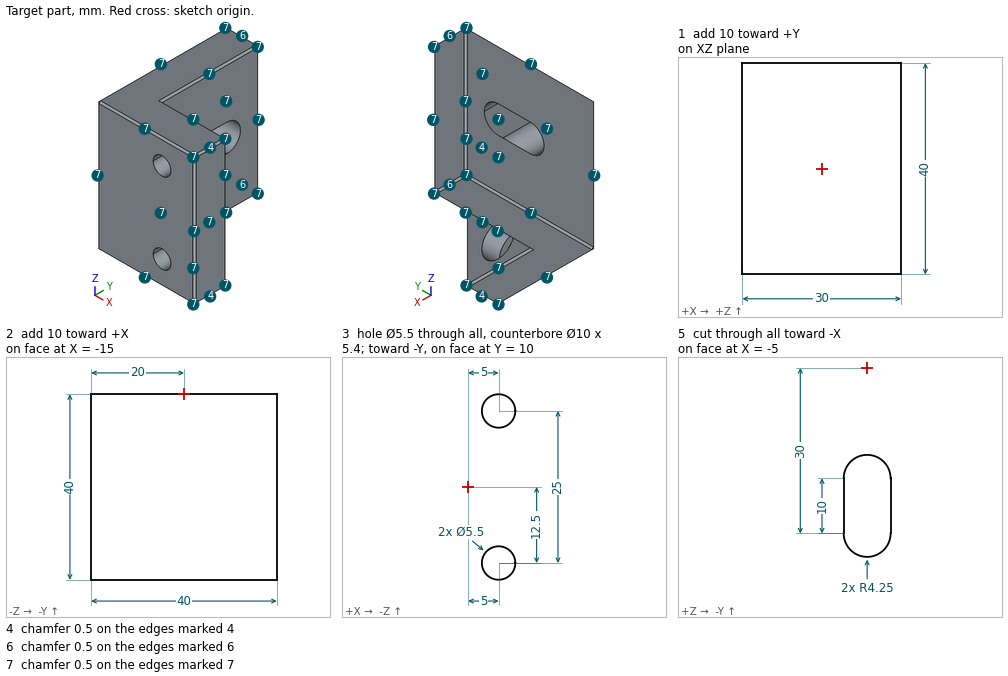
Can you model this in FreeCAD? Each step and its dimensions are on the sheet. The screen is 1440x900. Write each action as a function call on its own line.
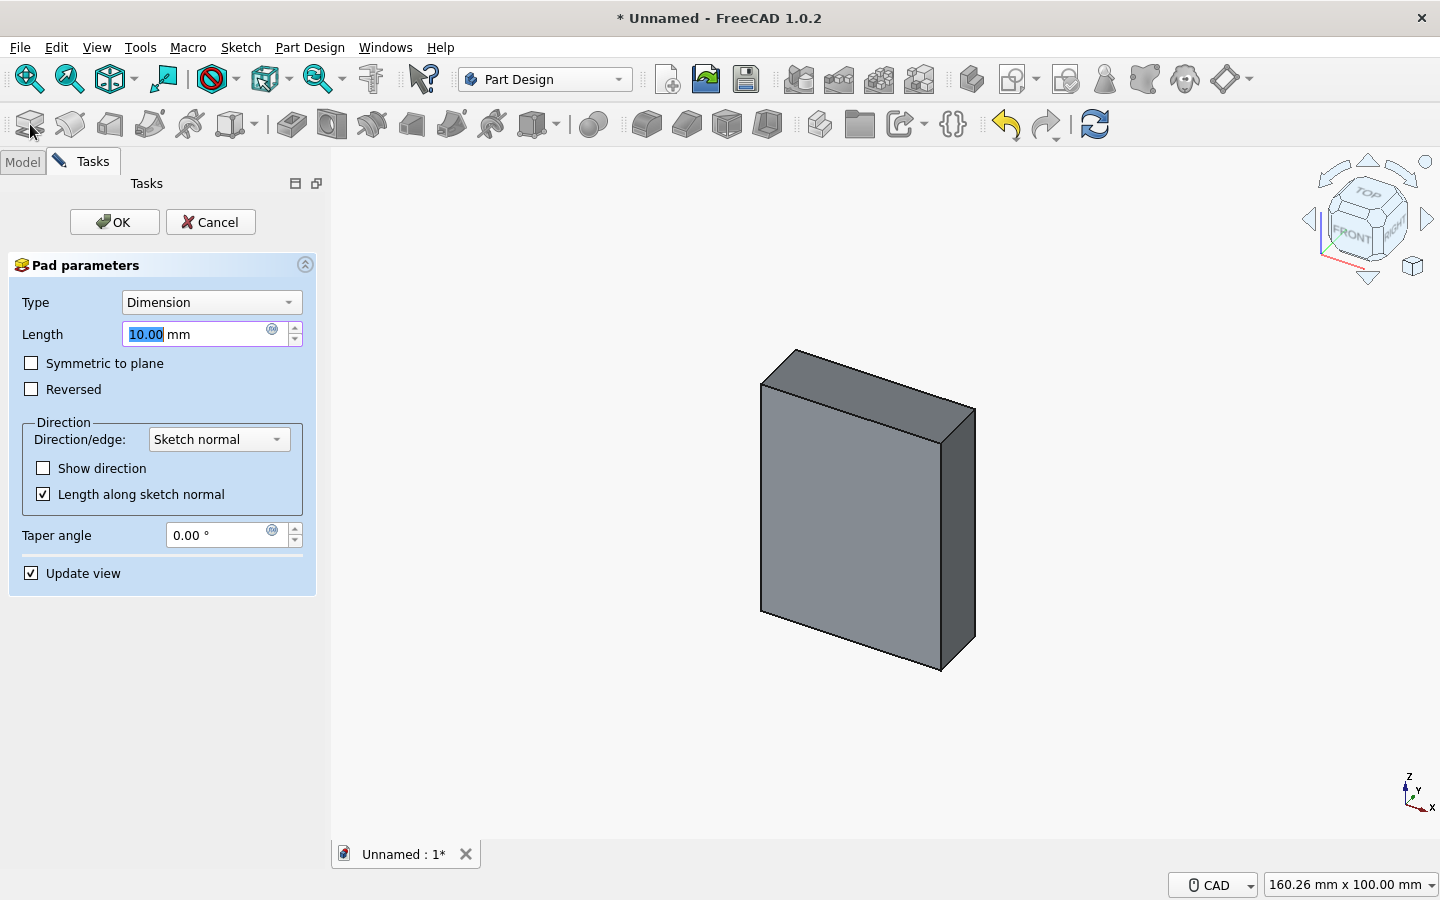
text(10)
key(Tab)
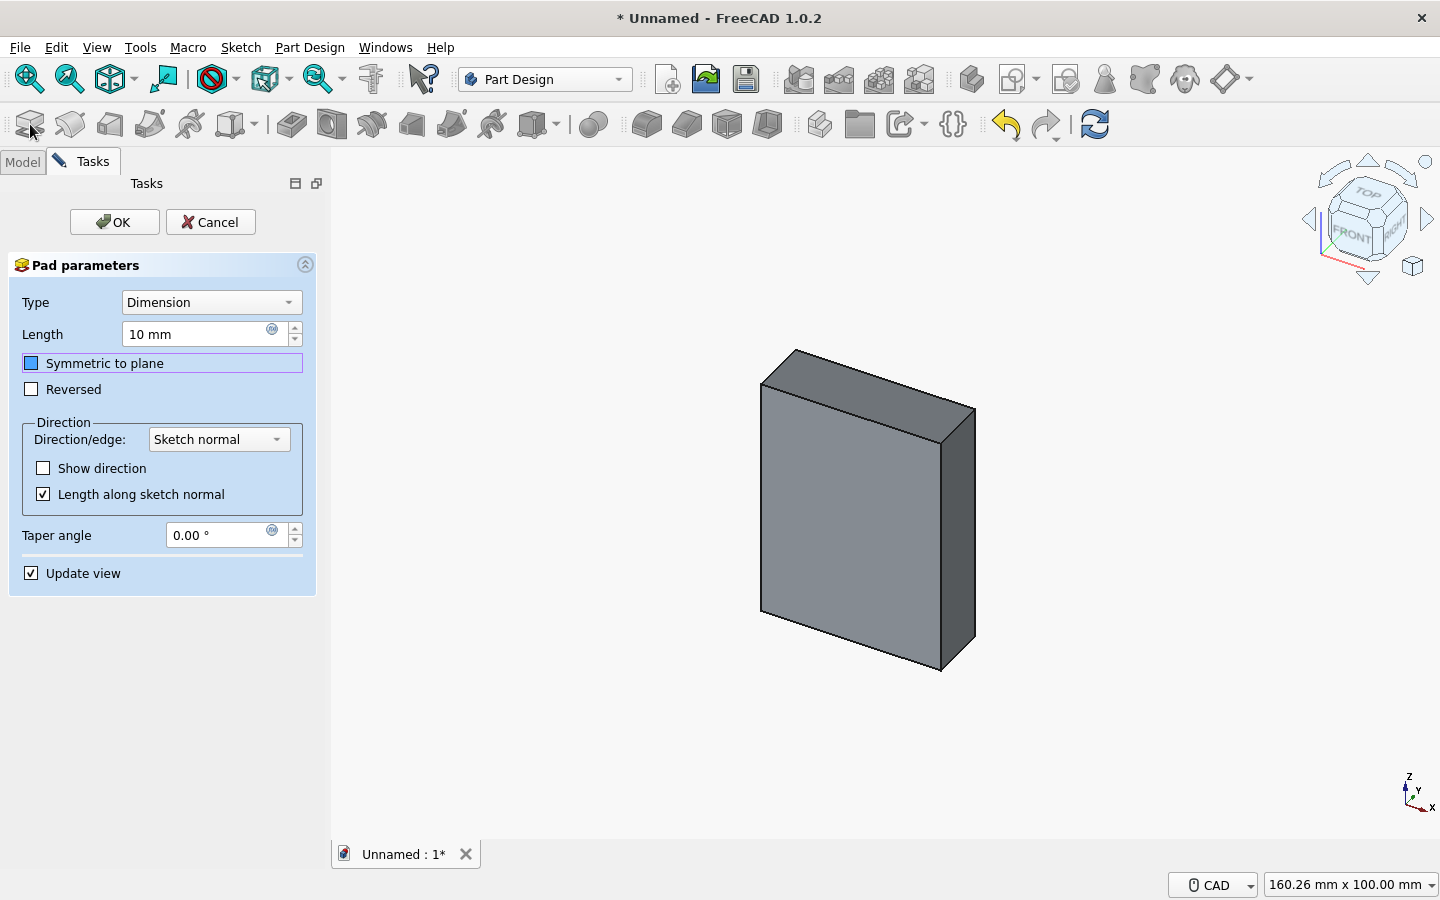
click(30, 389)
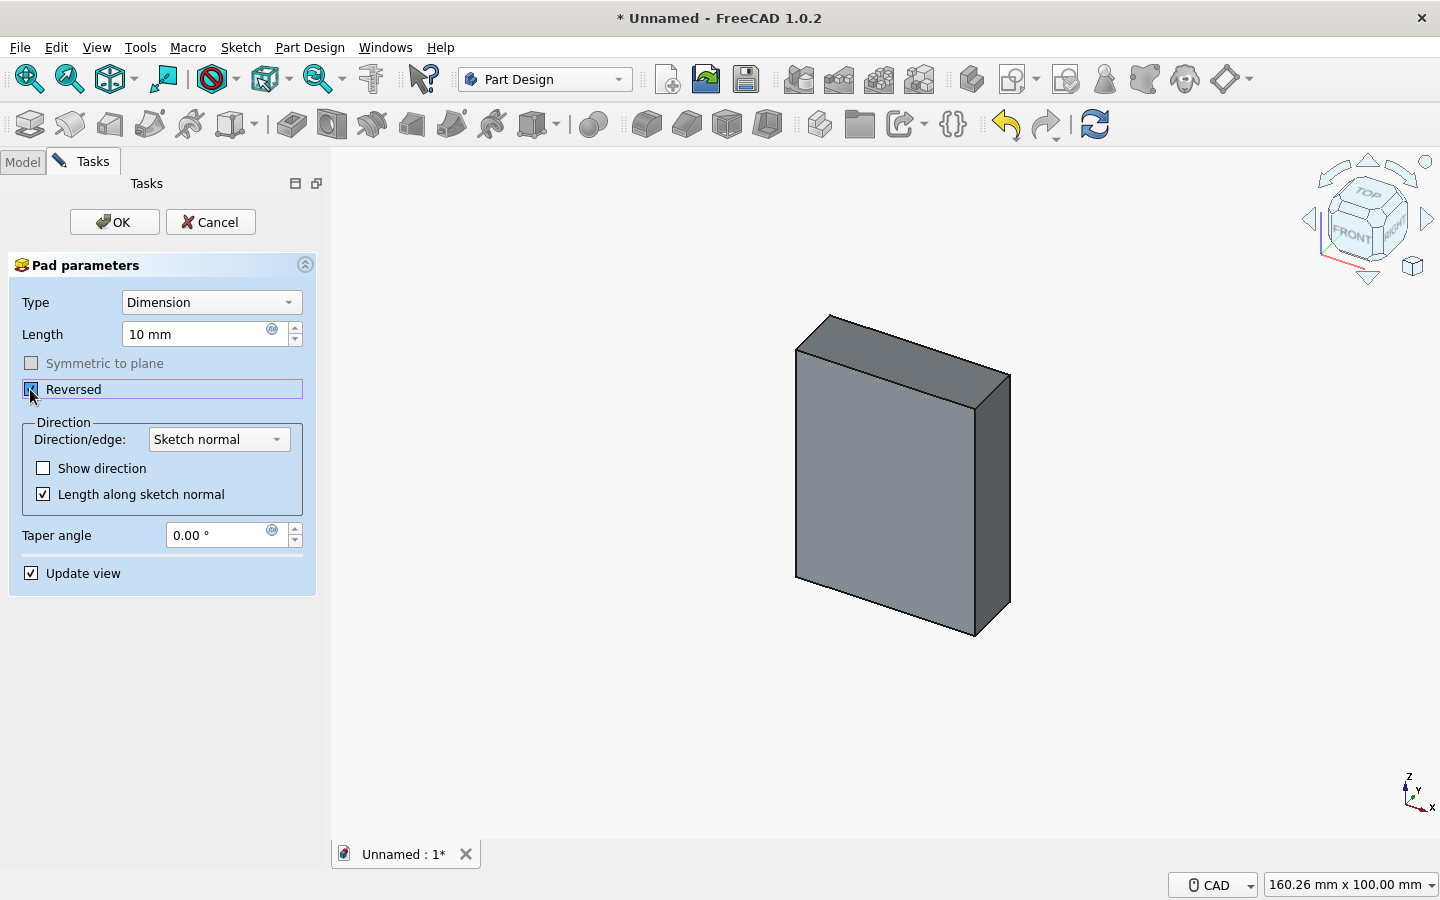
click(115, 222)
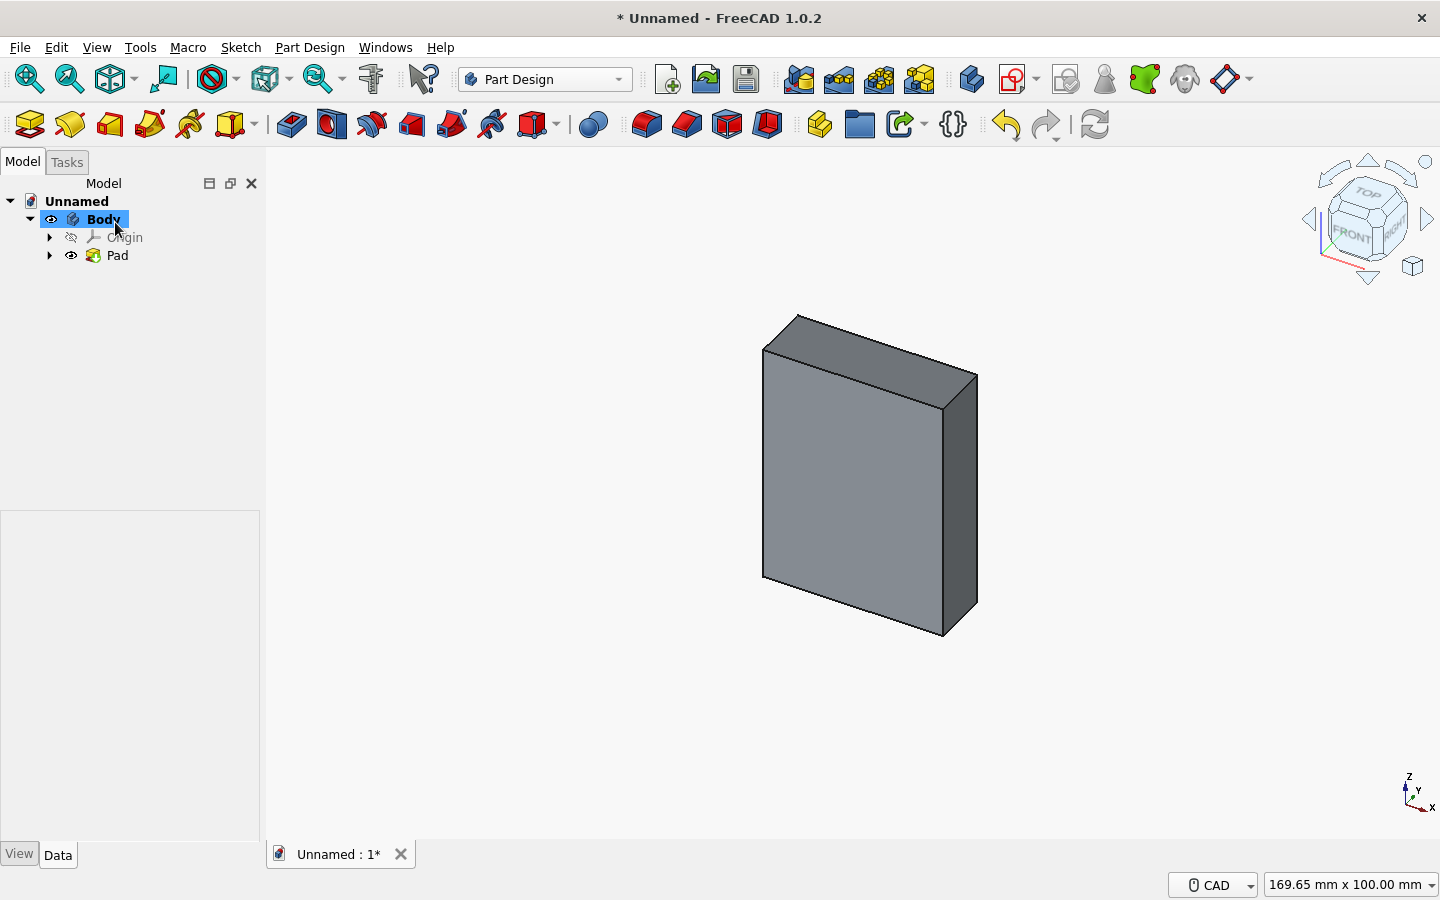
key(6)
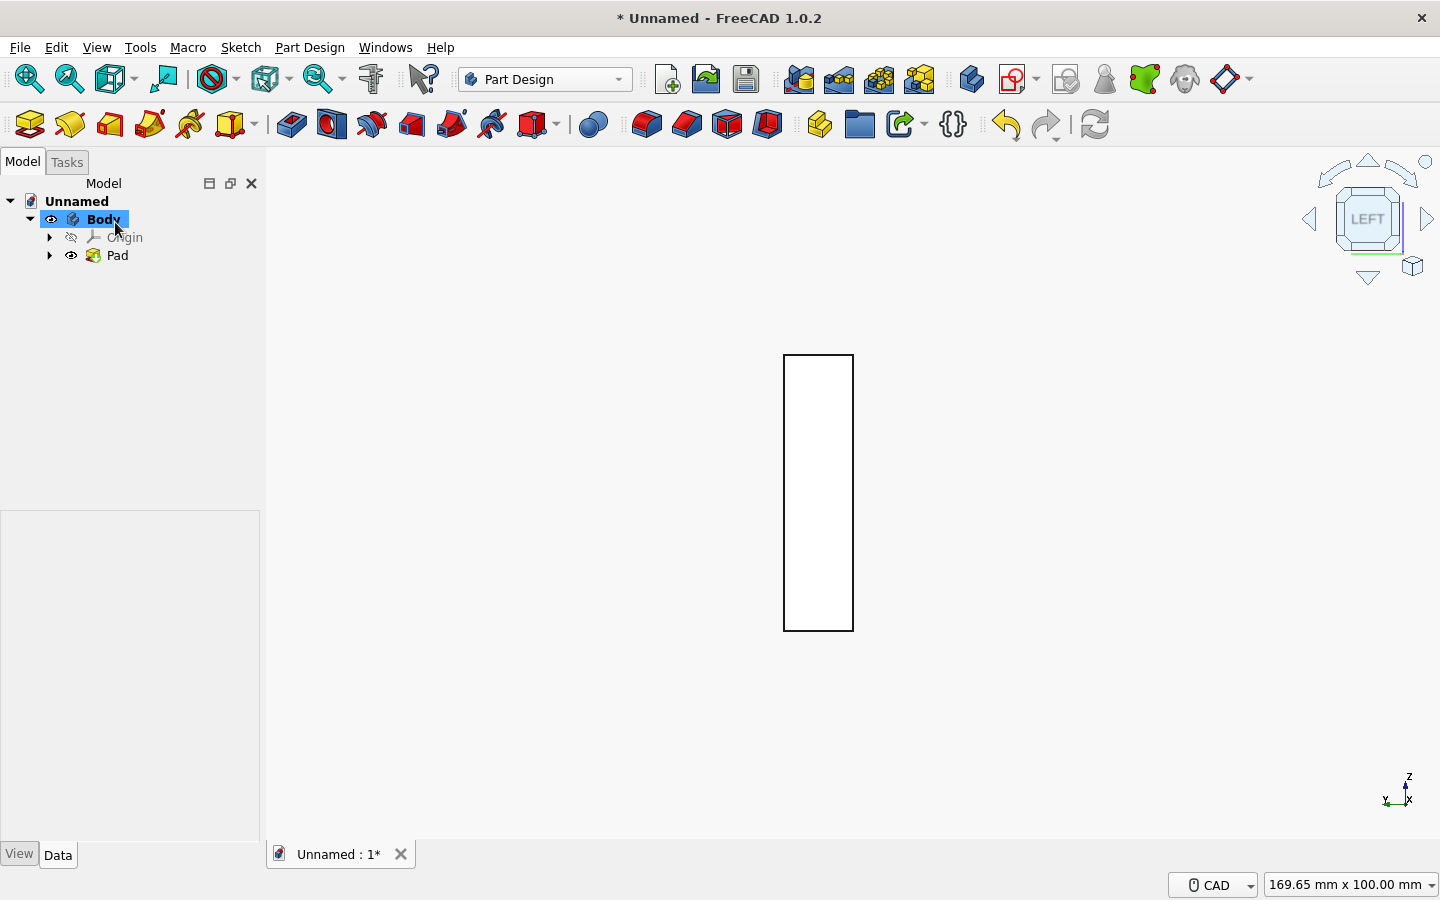
click(30, 80)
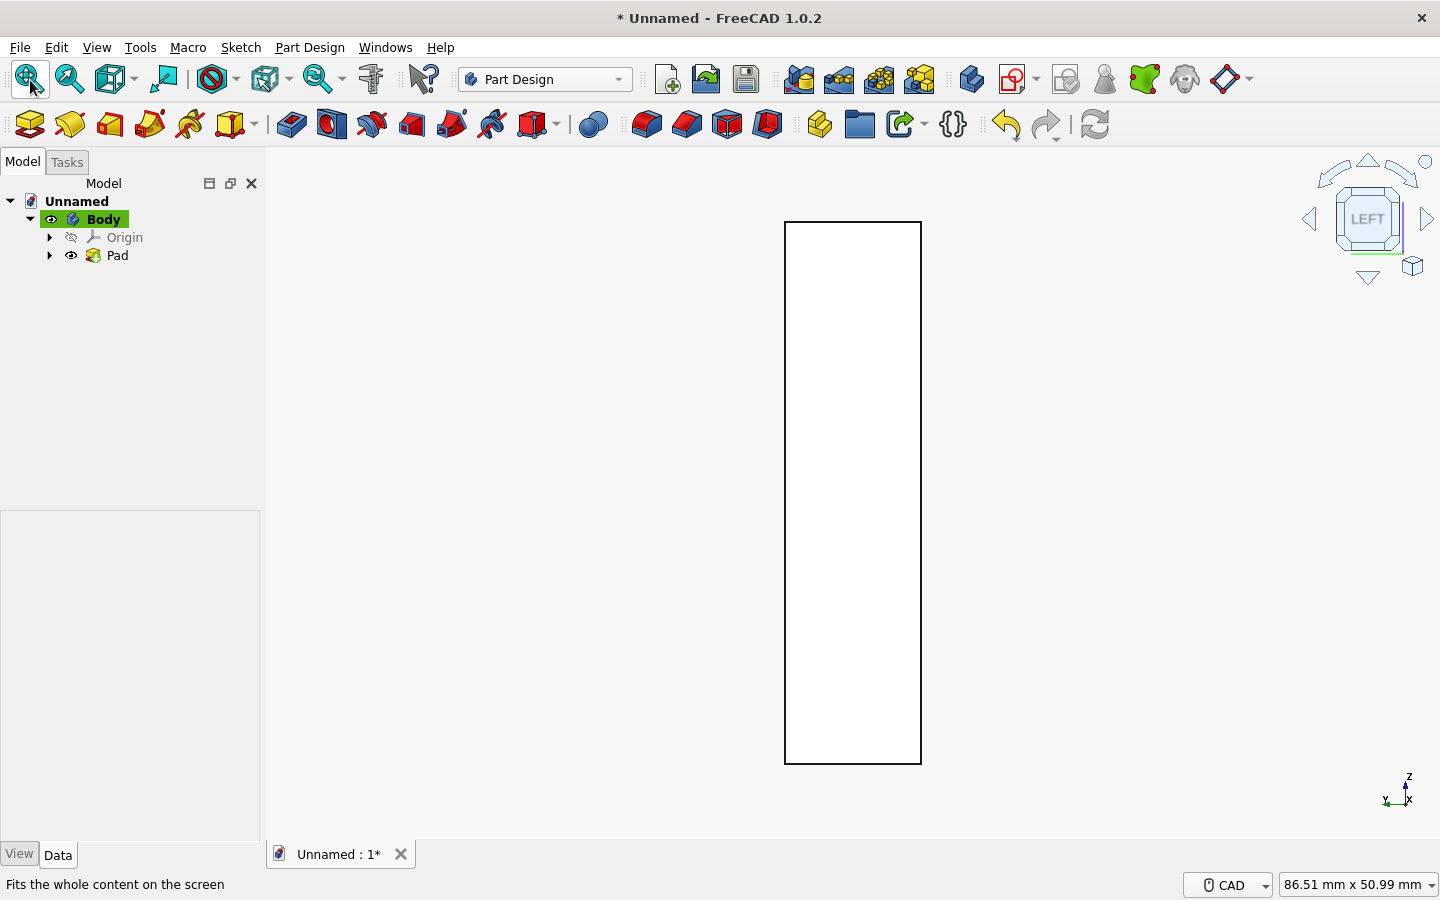
click(853, 337)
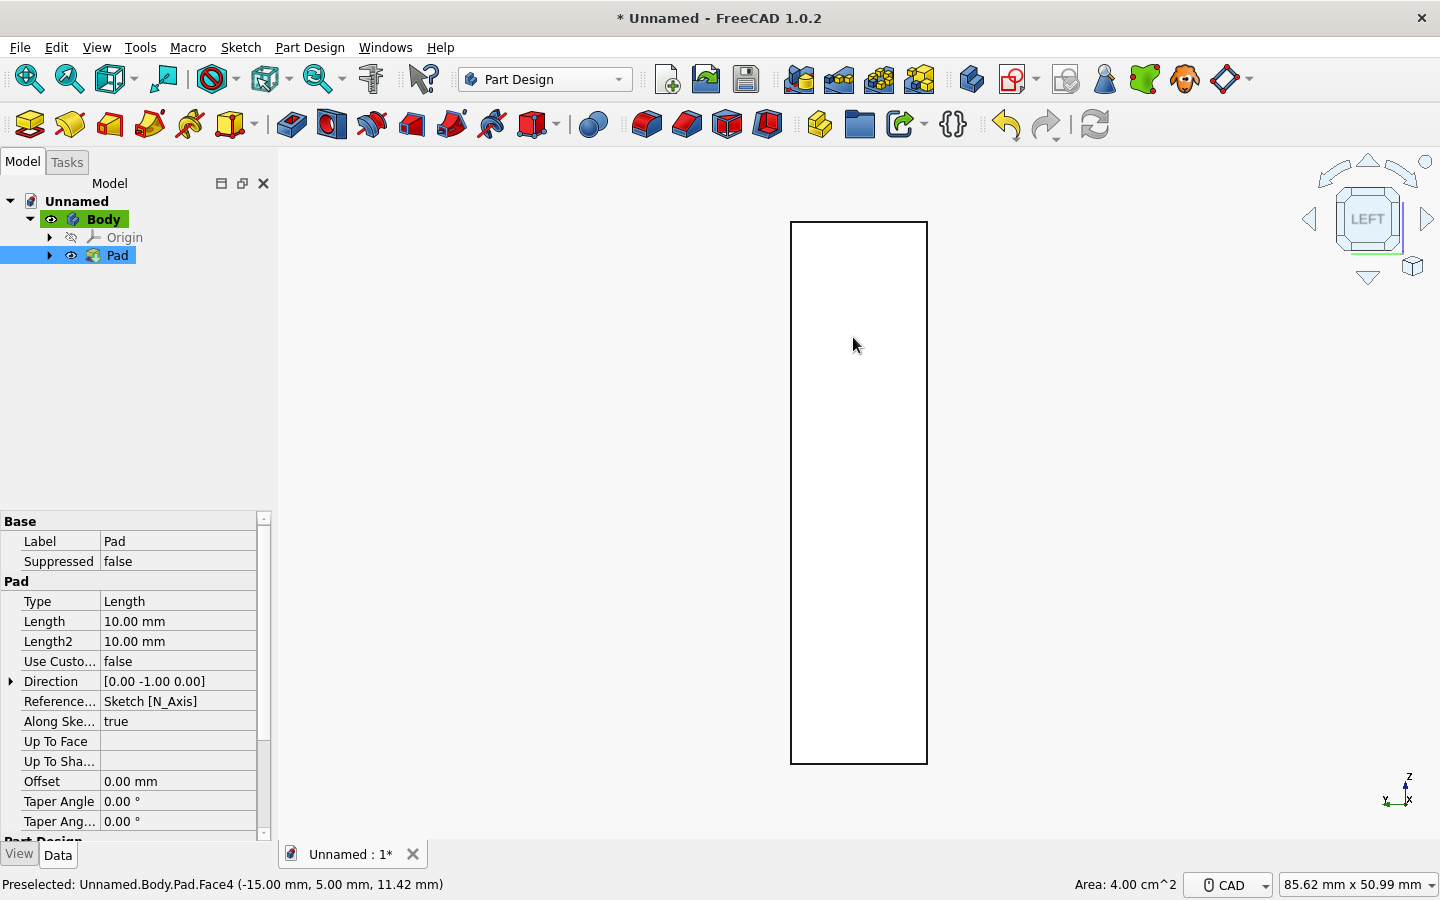
click(1012, 80)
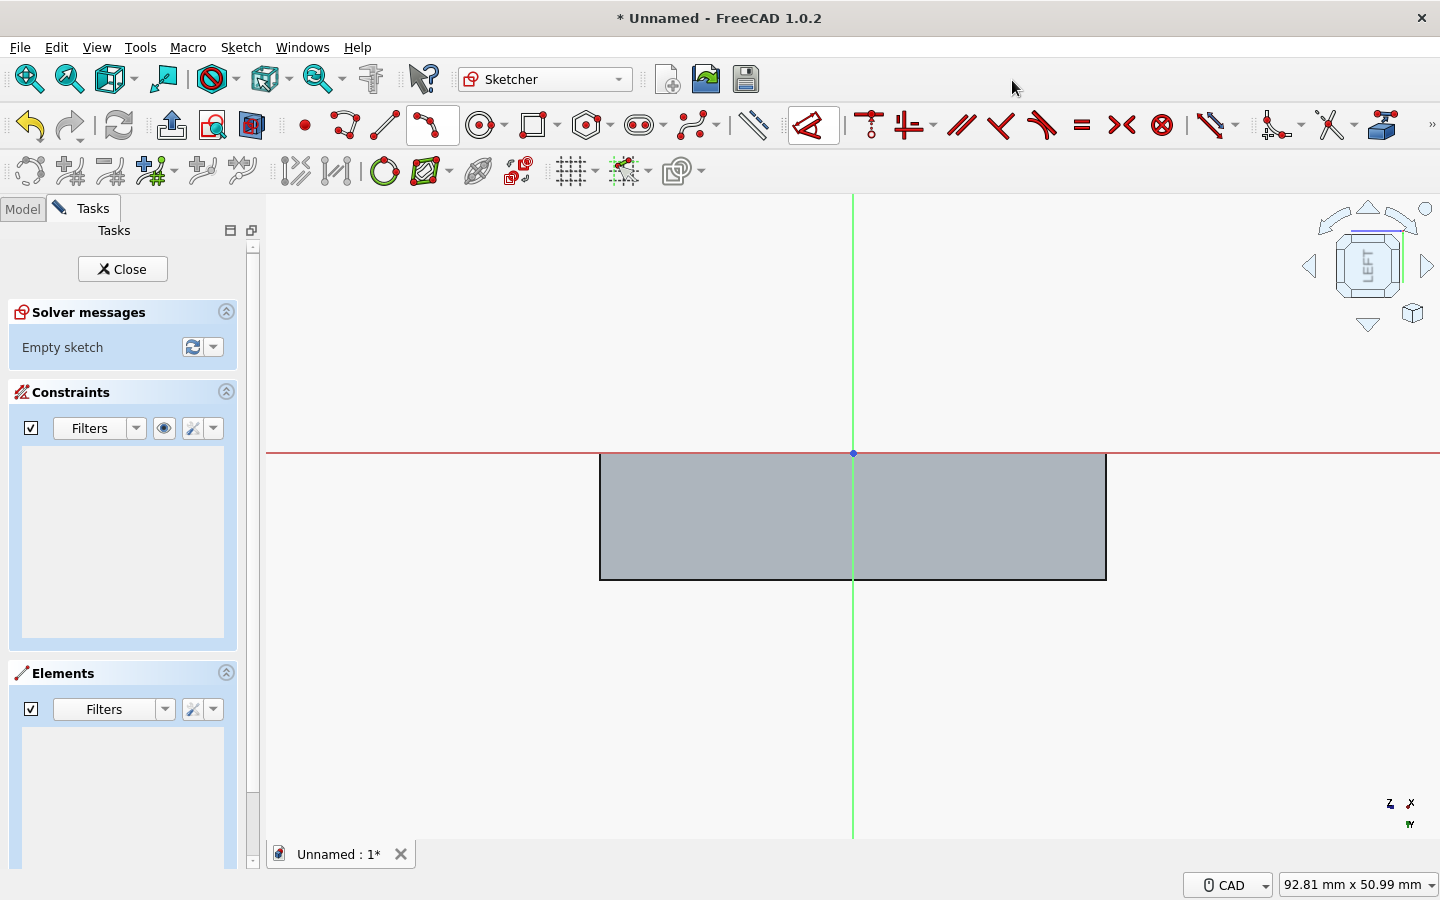
scroll(645, 222, down, 2)